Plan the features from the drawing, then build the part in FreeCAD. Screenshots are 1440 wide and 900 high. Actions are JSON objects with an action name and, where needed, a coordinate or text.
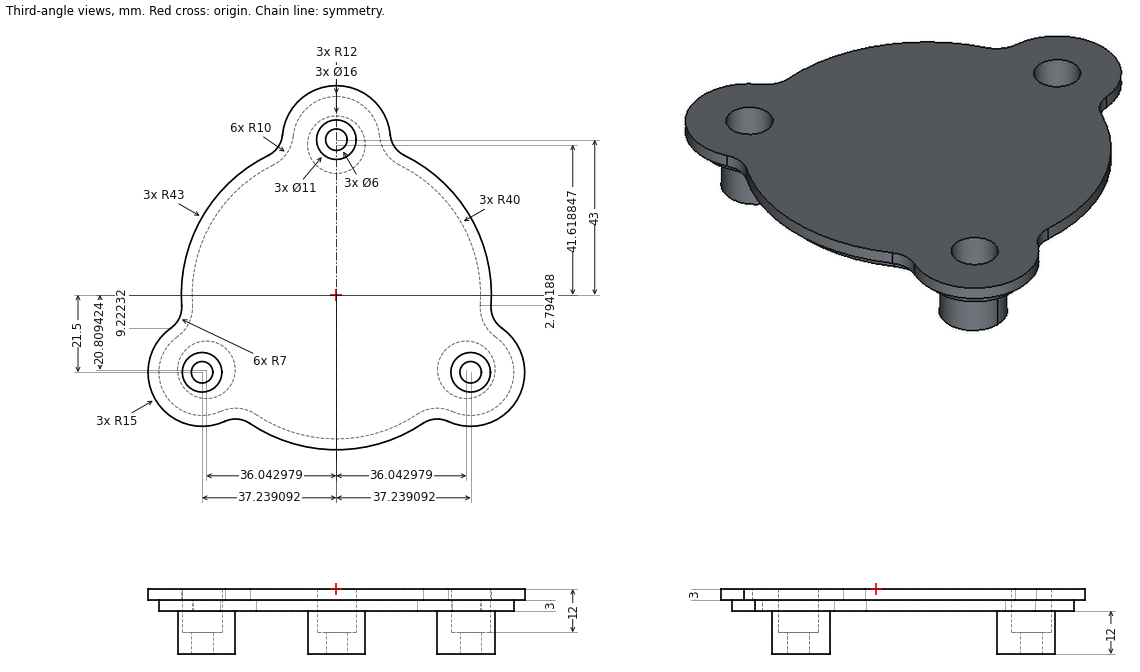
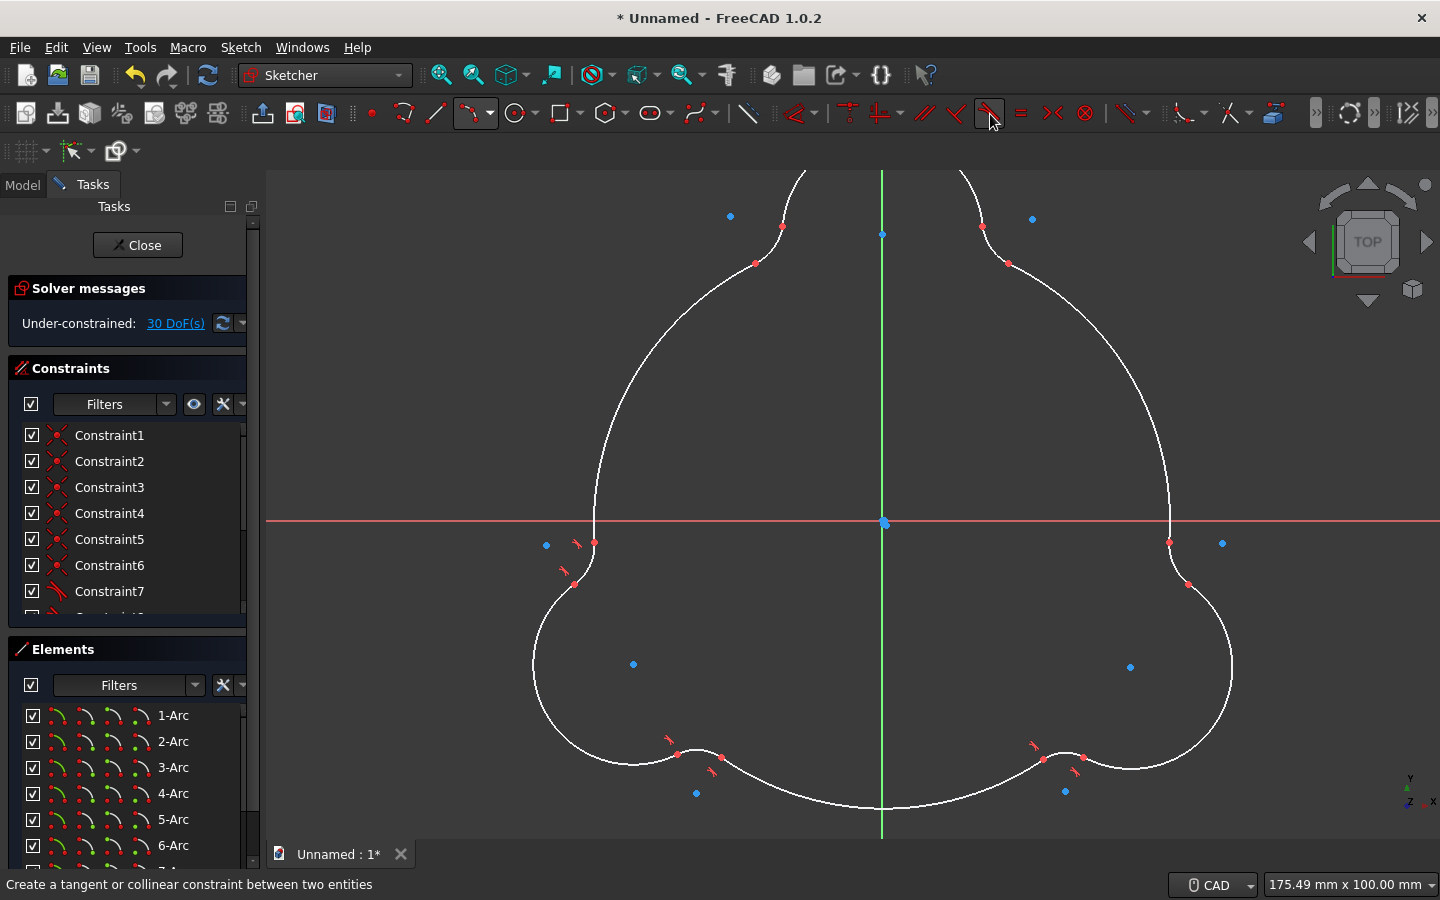
{"action": "left_click", "coordinate": [1172, 760]}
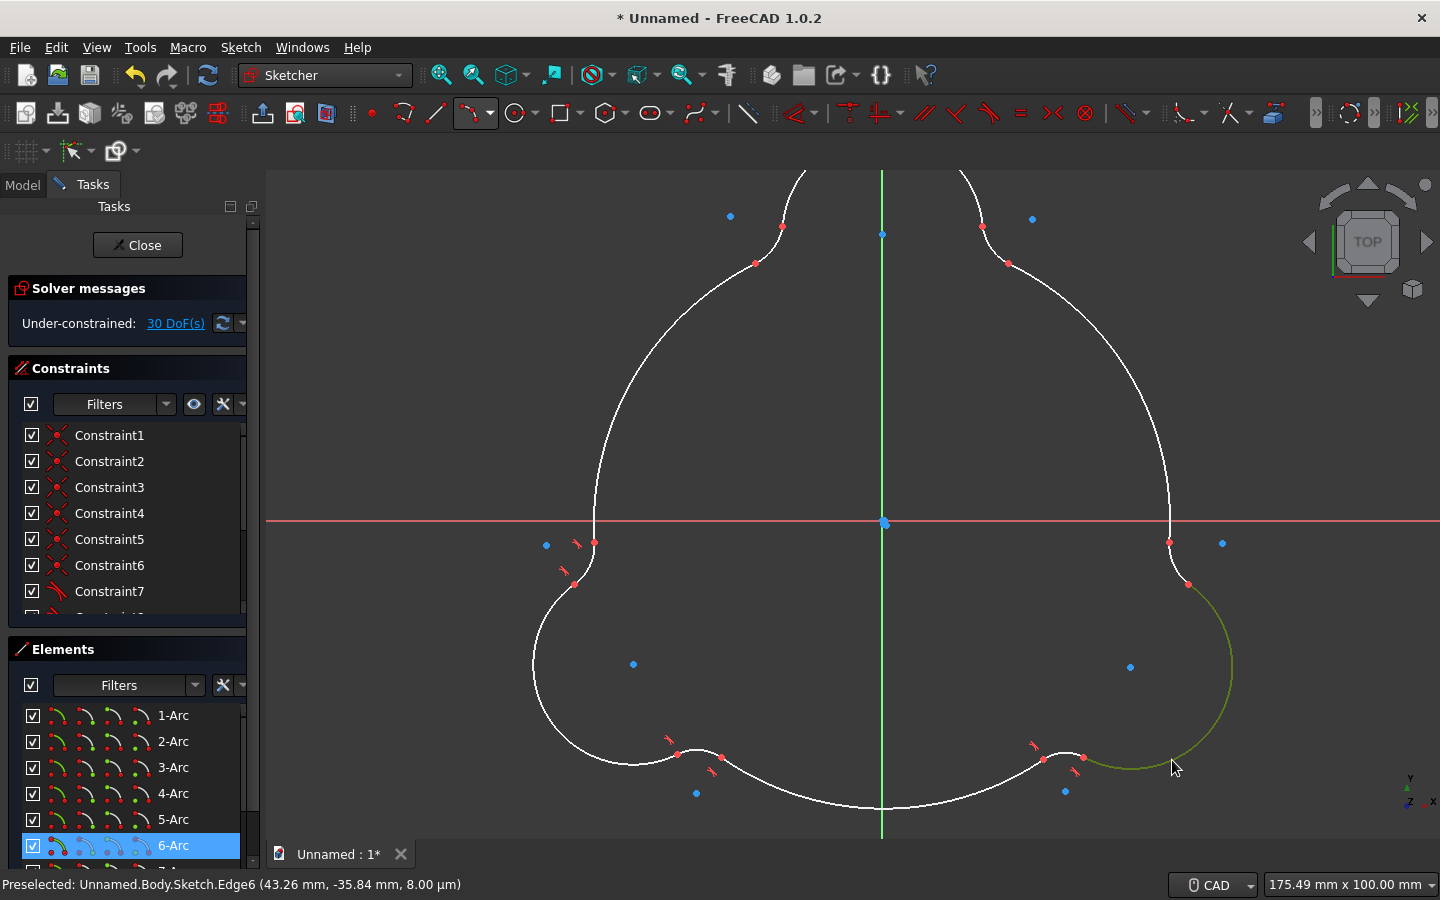
{"action": "left_click", "coordinate": [1171, 557]}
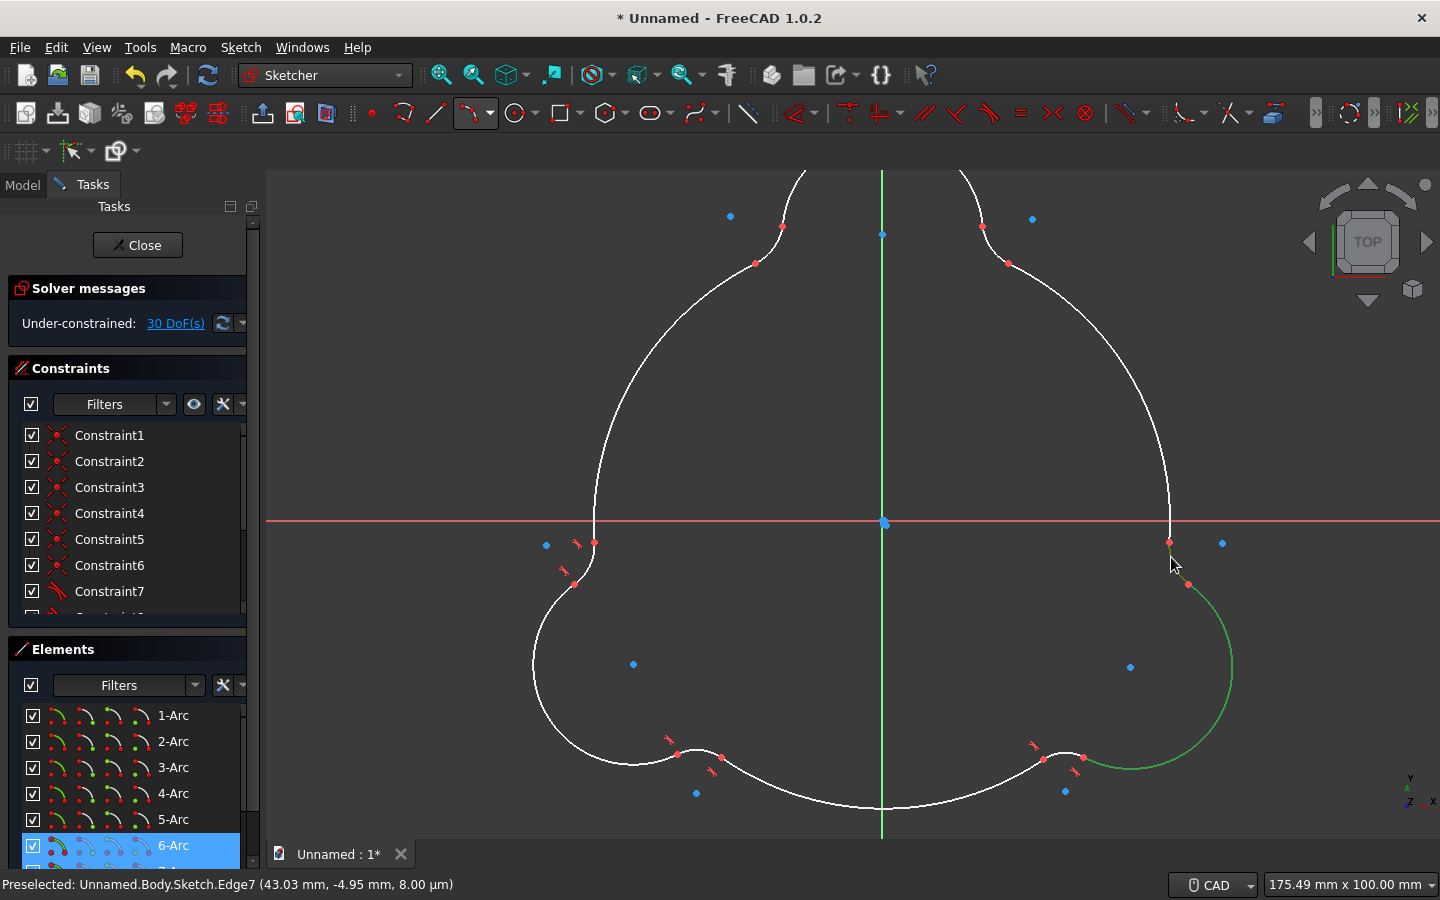
{"action": "left_click", "coordinate": [990, 114]}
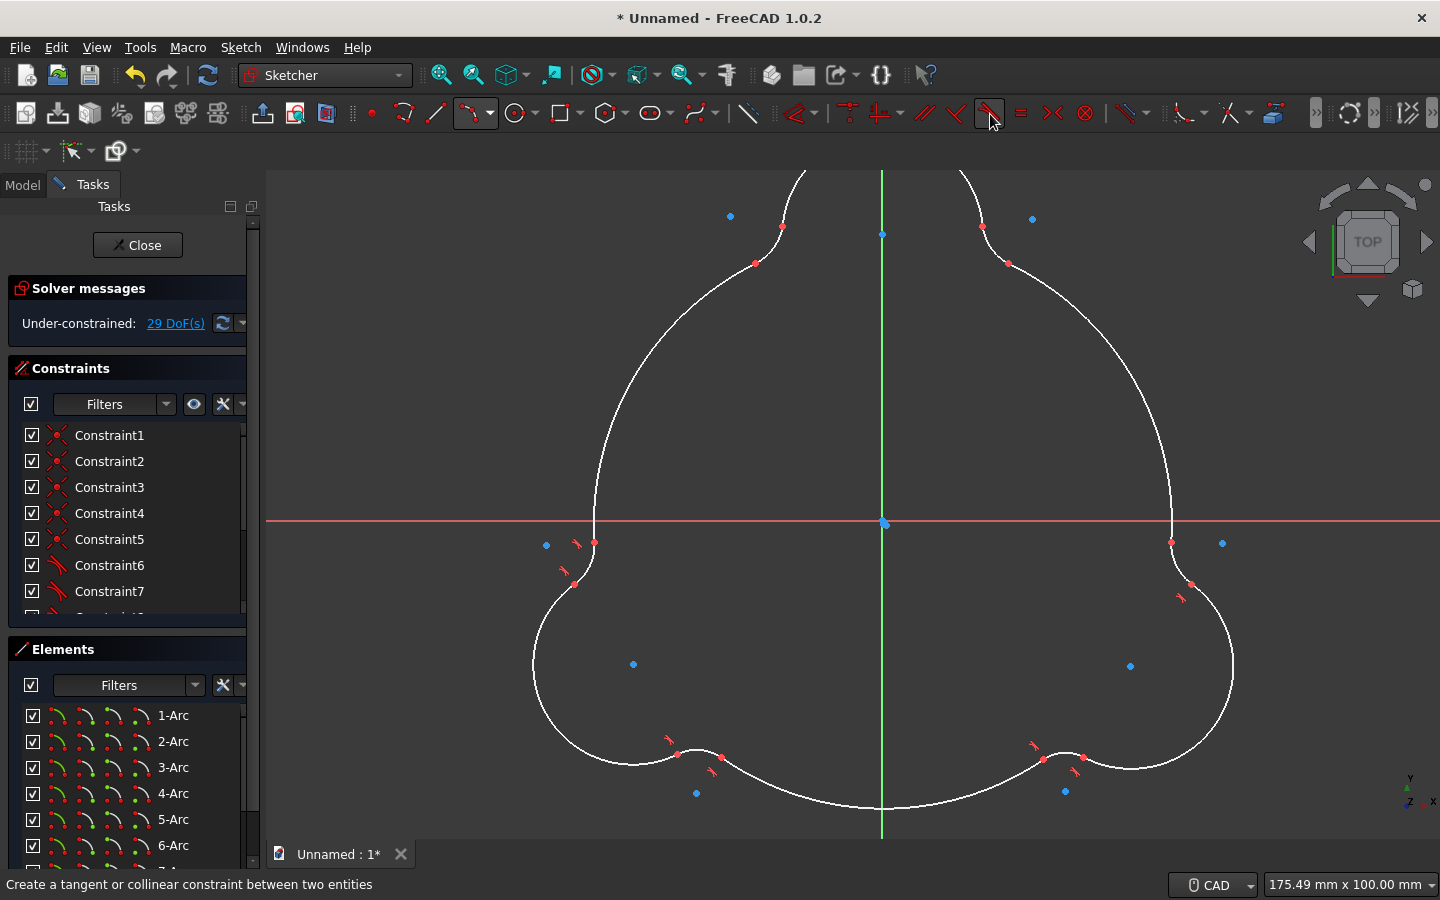
{"action": "left_click", "coordinate": [1173, 557]}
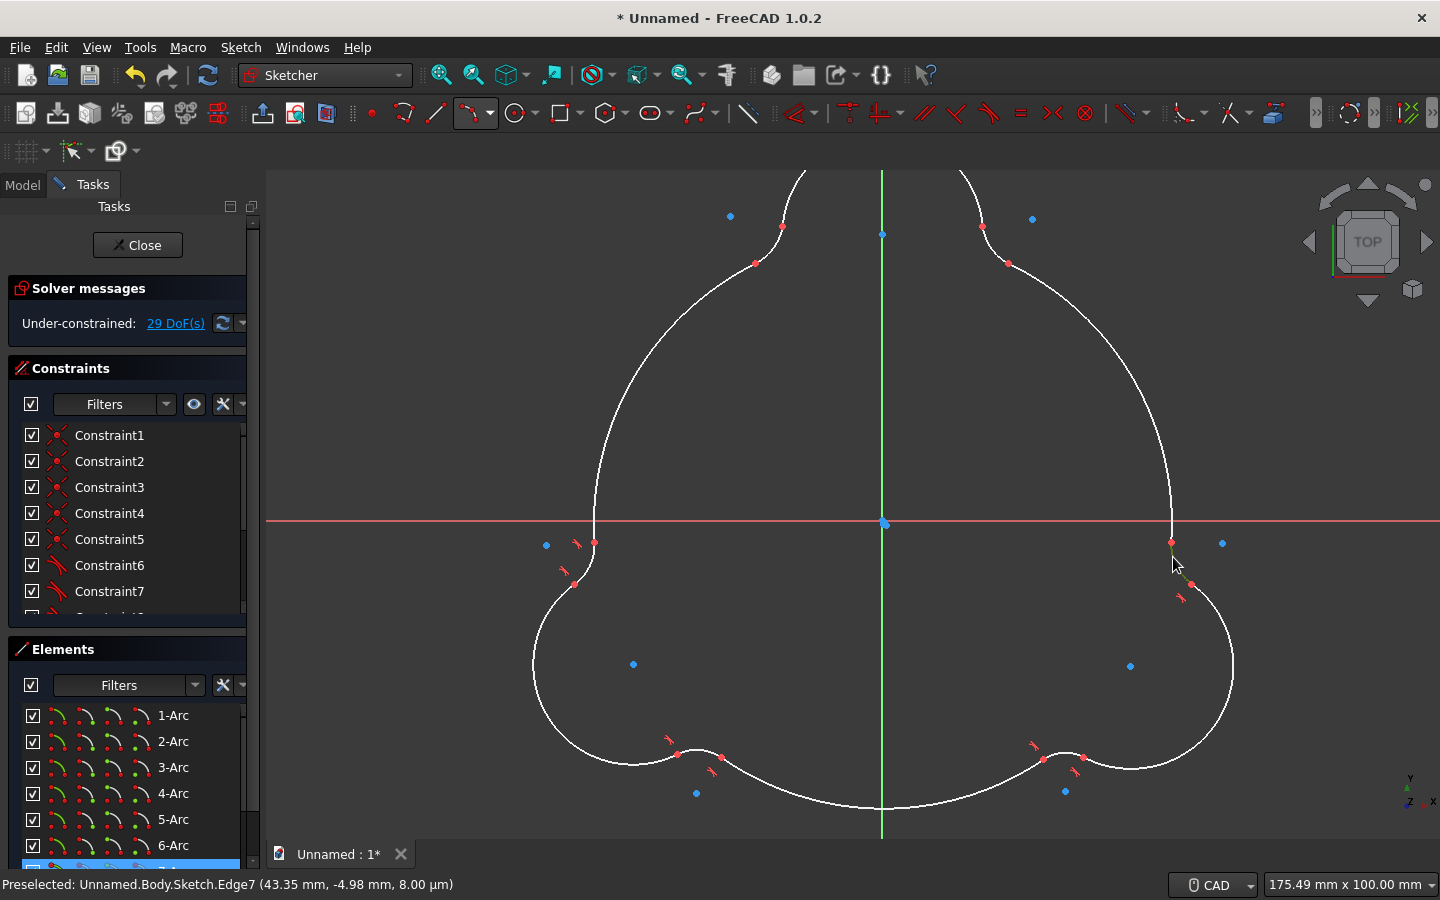
{"action": "left_click", "coordinate": [1160, 441]}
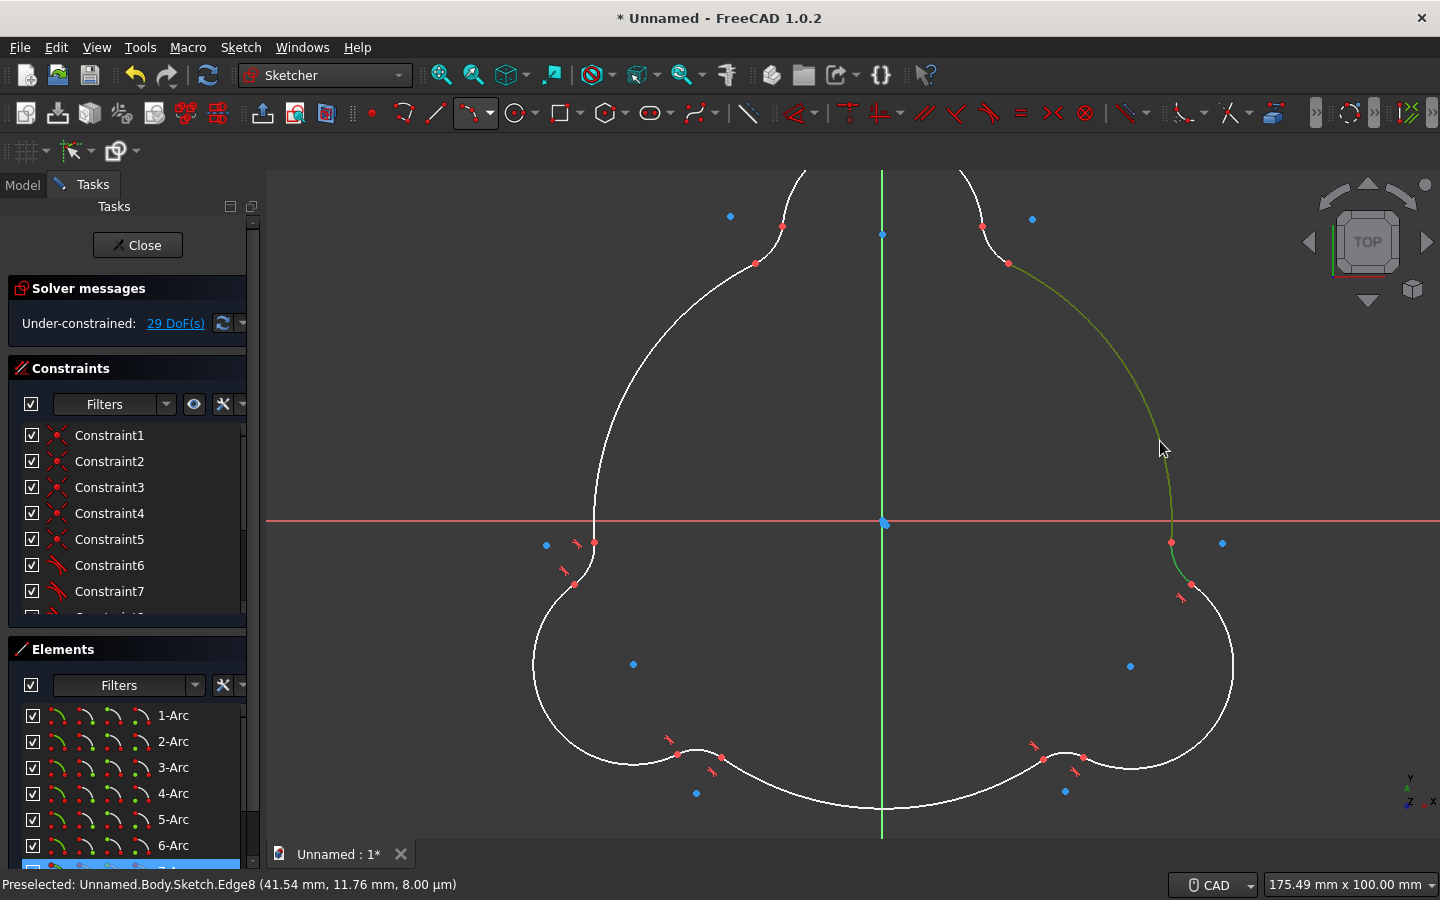
{"action": "left_click", "coordinate": [990, 114]}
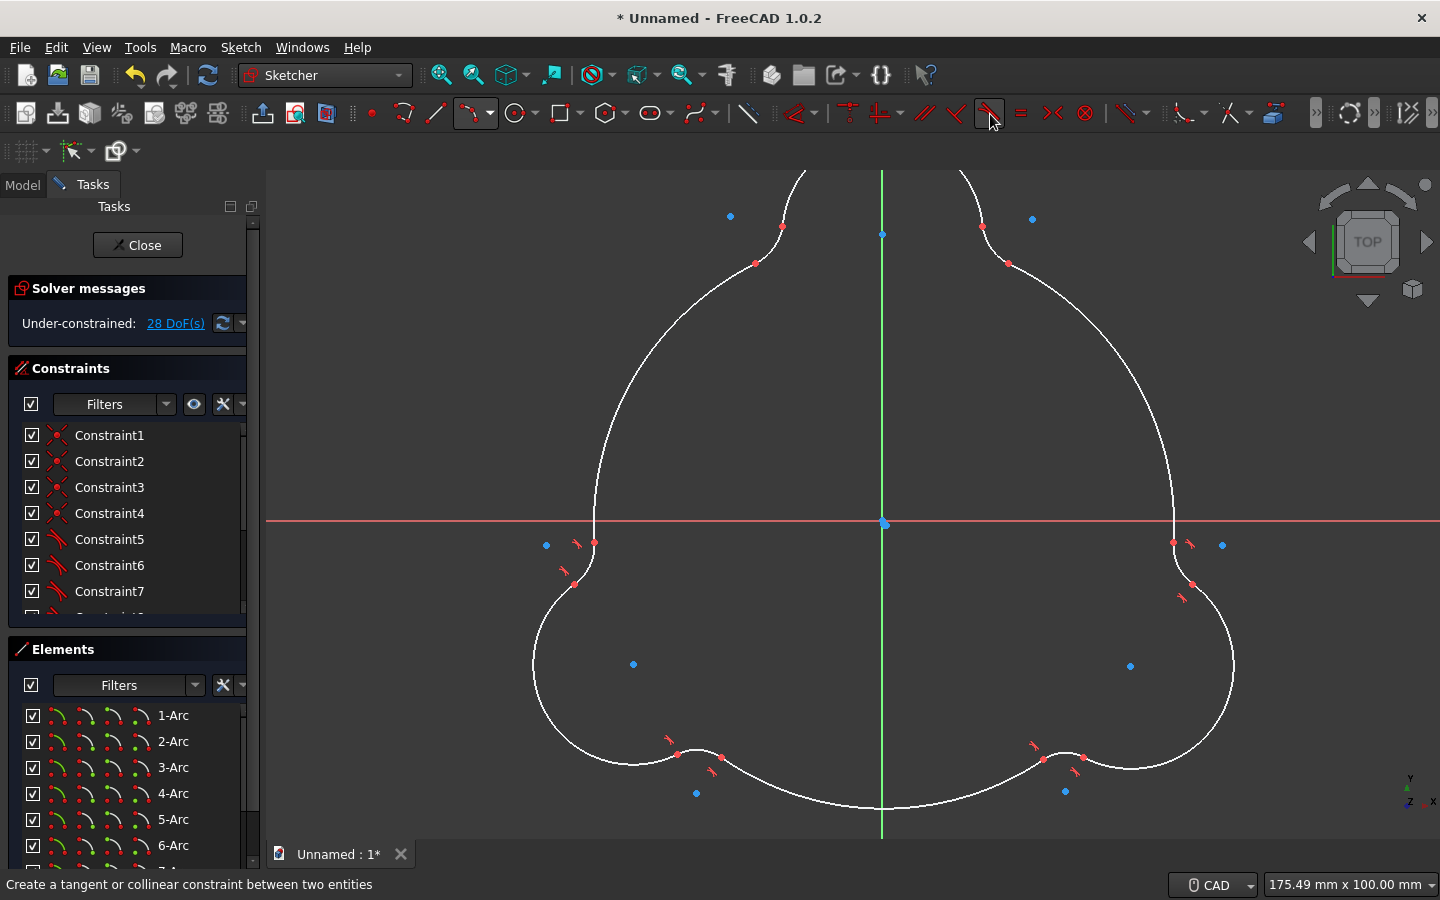
{"action": "left_click", "coordinate": [1161, 440]}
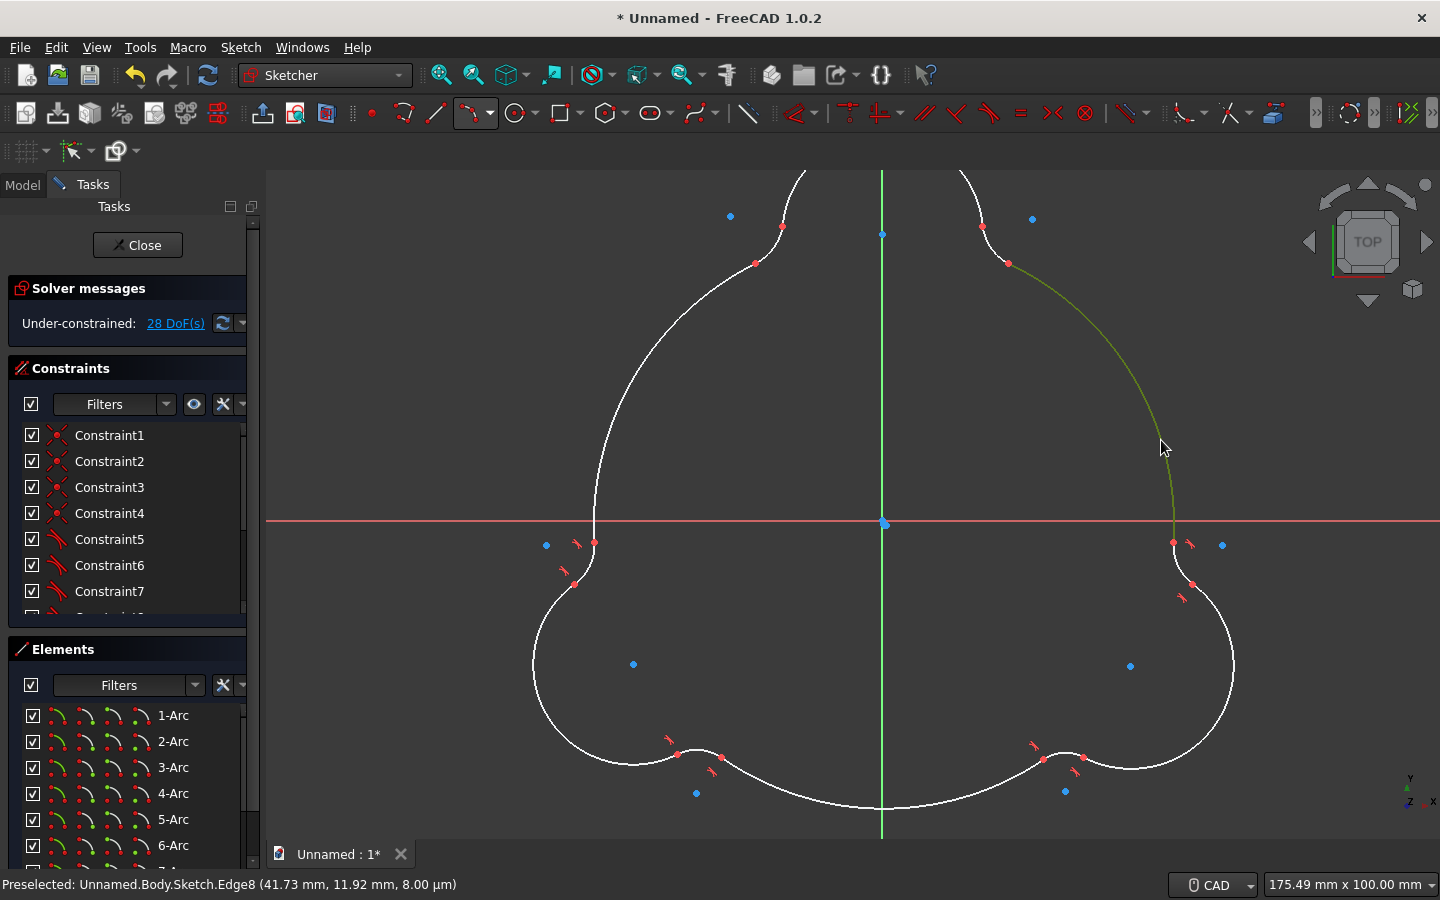
{"action": "left_click", "coordinate": [986, 240]}